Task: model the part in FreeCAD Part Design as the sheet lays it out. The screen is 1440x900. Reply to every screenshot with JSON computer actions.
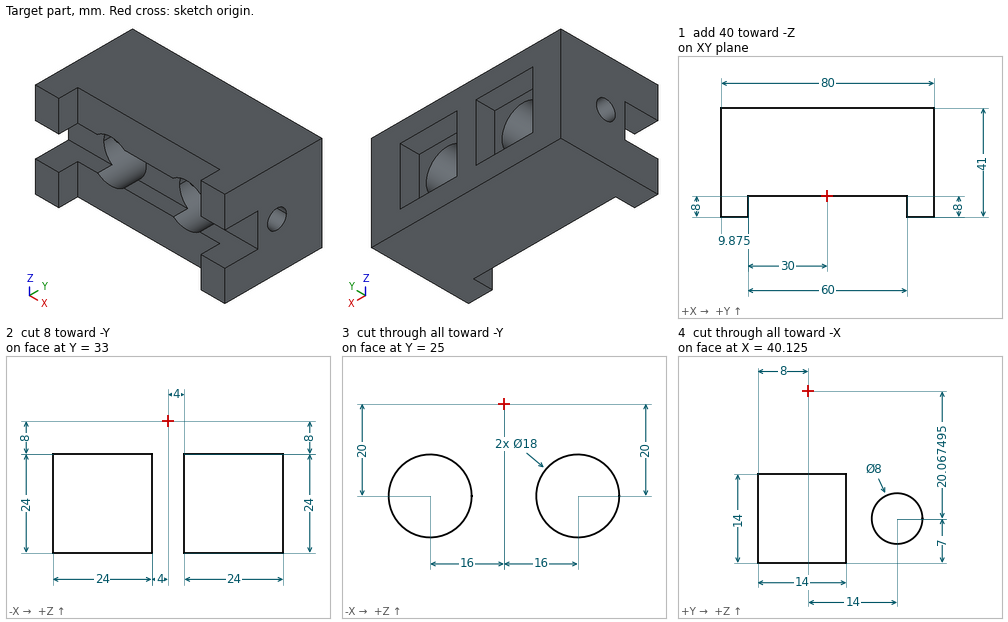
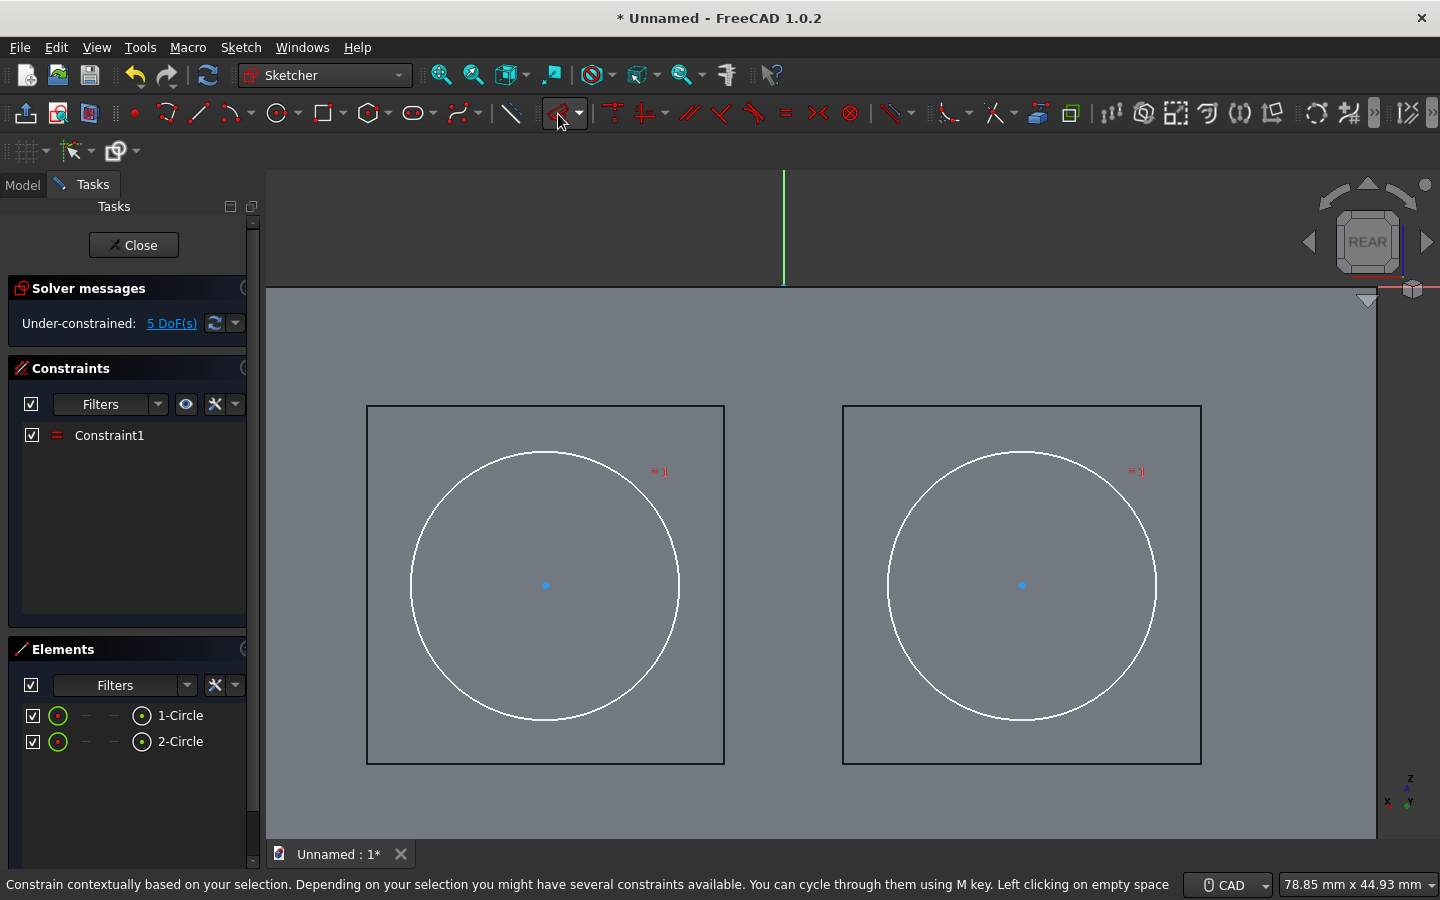
{"action": "left_click", "coordinate": [1117, 491]}
{"action": "left_click", "coordinate": [1140, 468]}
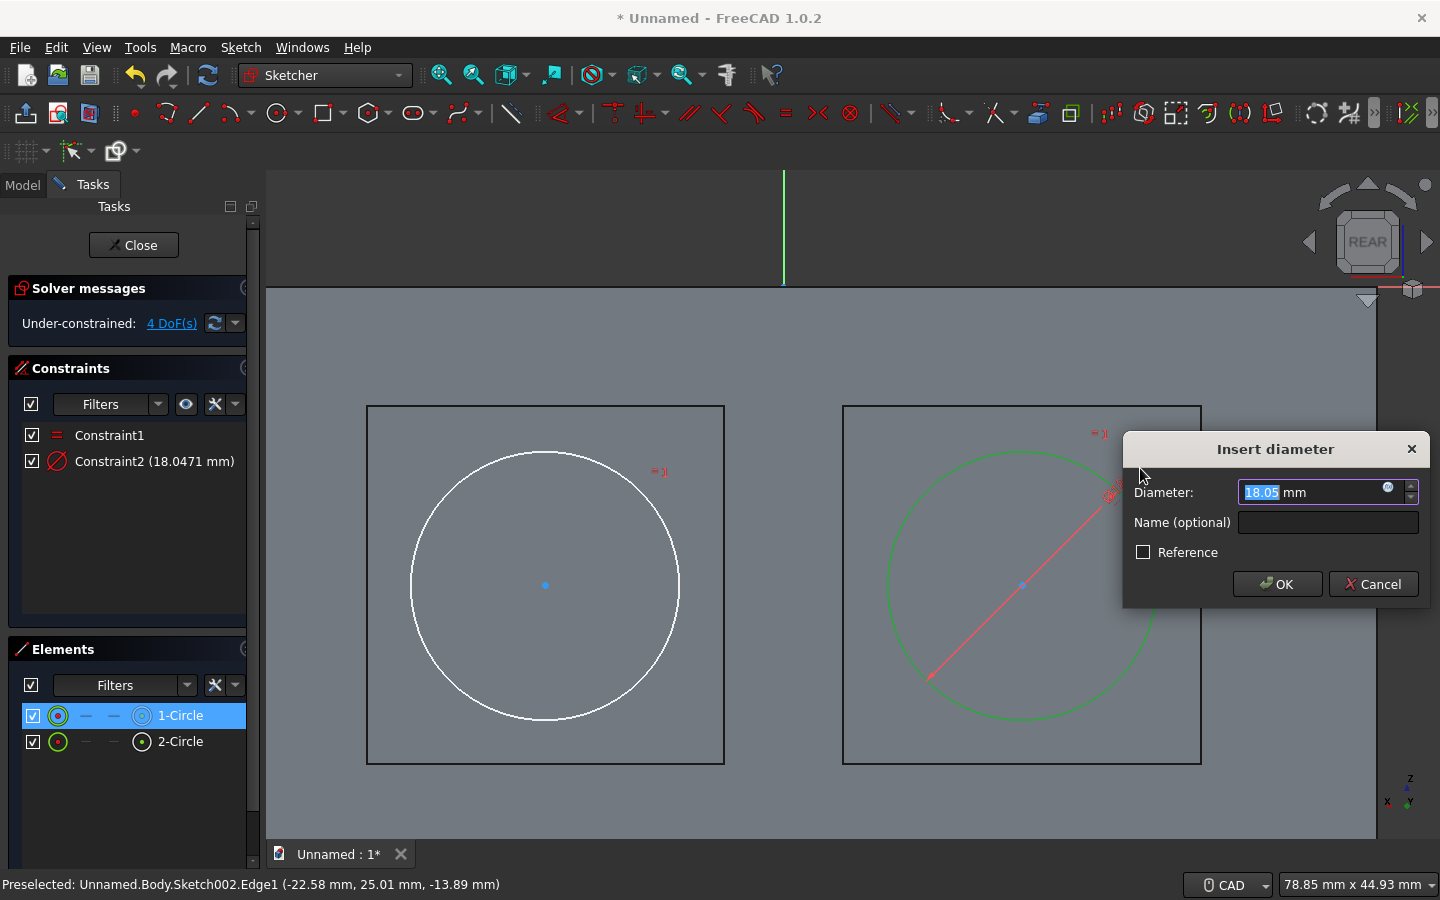
{"action": "type", "text": "18"}
{"action": "key", "text": "Return"}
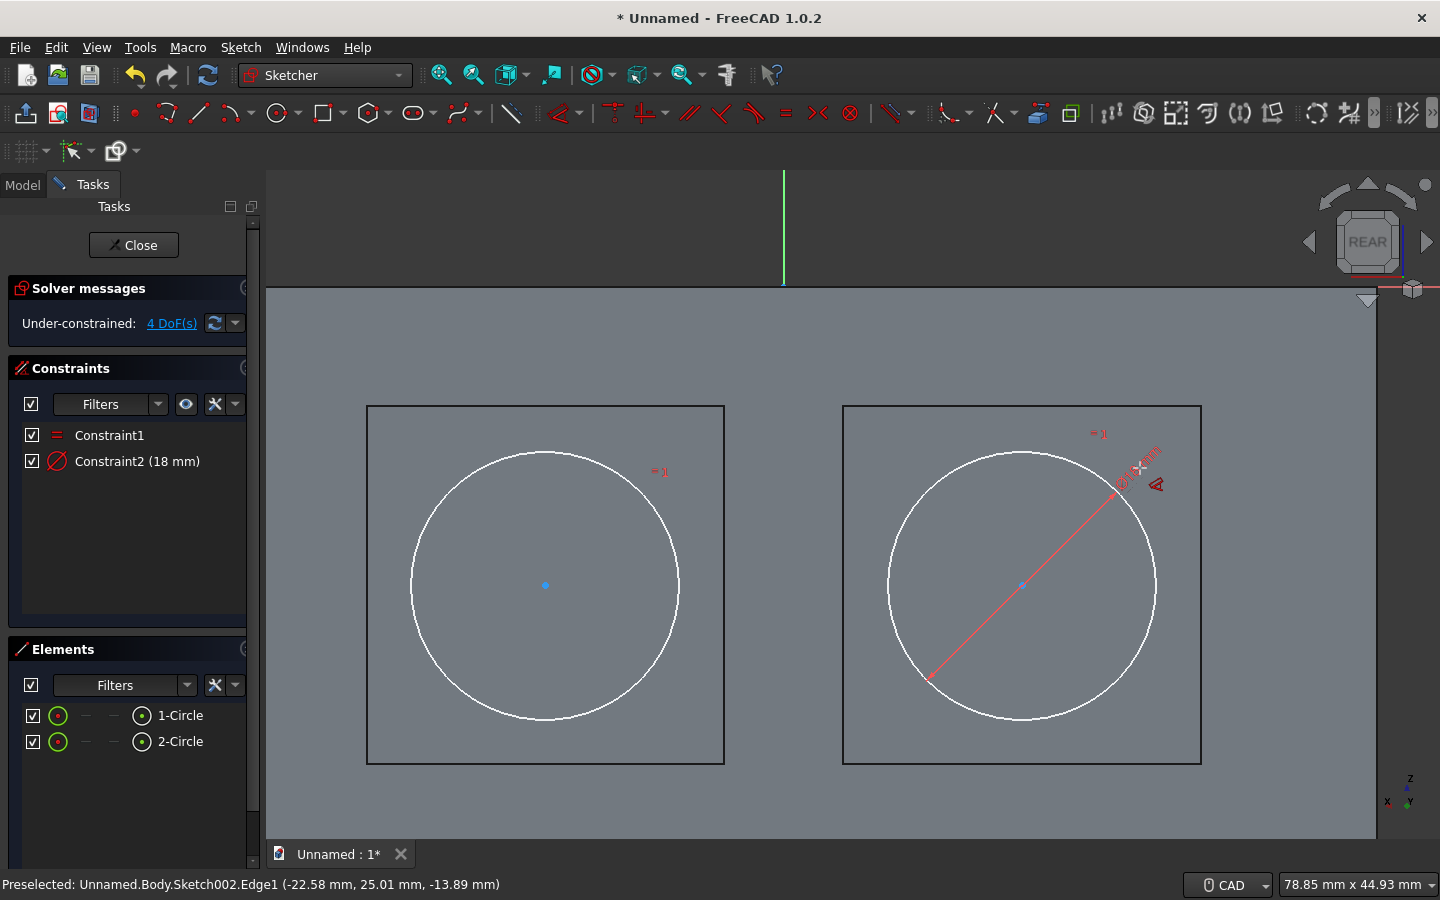
{"action": "left_click", "coordinate": [1022, 586]}
{"action": "left_click", "coordinate": [903, 253]}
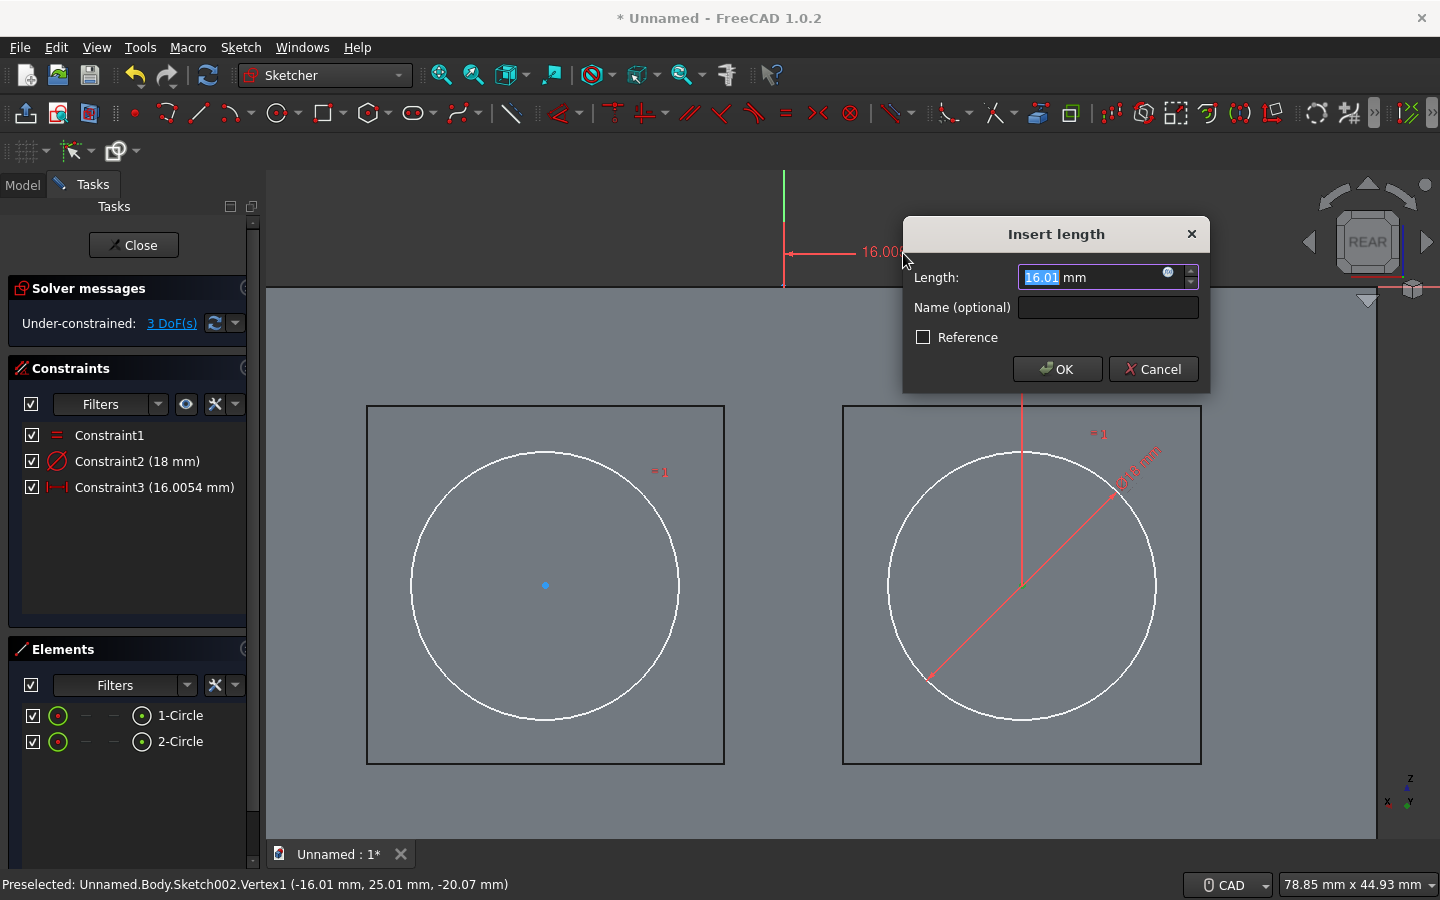
{"action": "type", "text": "16"}
{"action": "key", "text": "Return"}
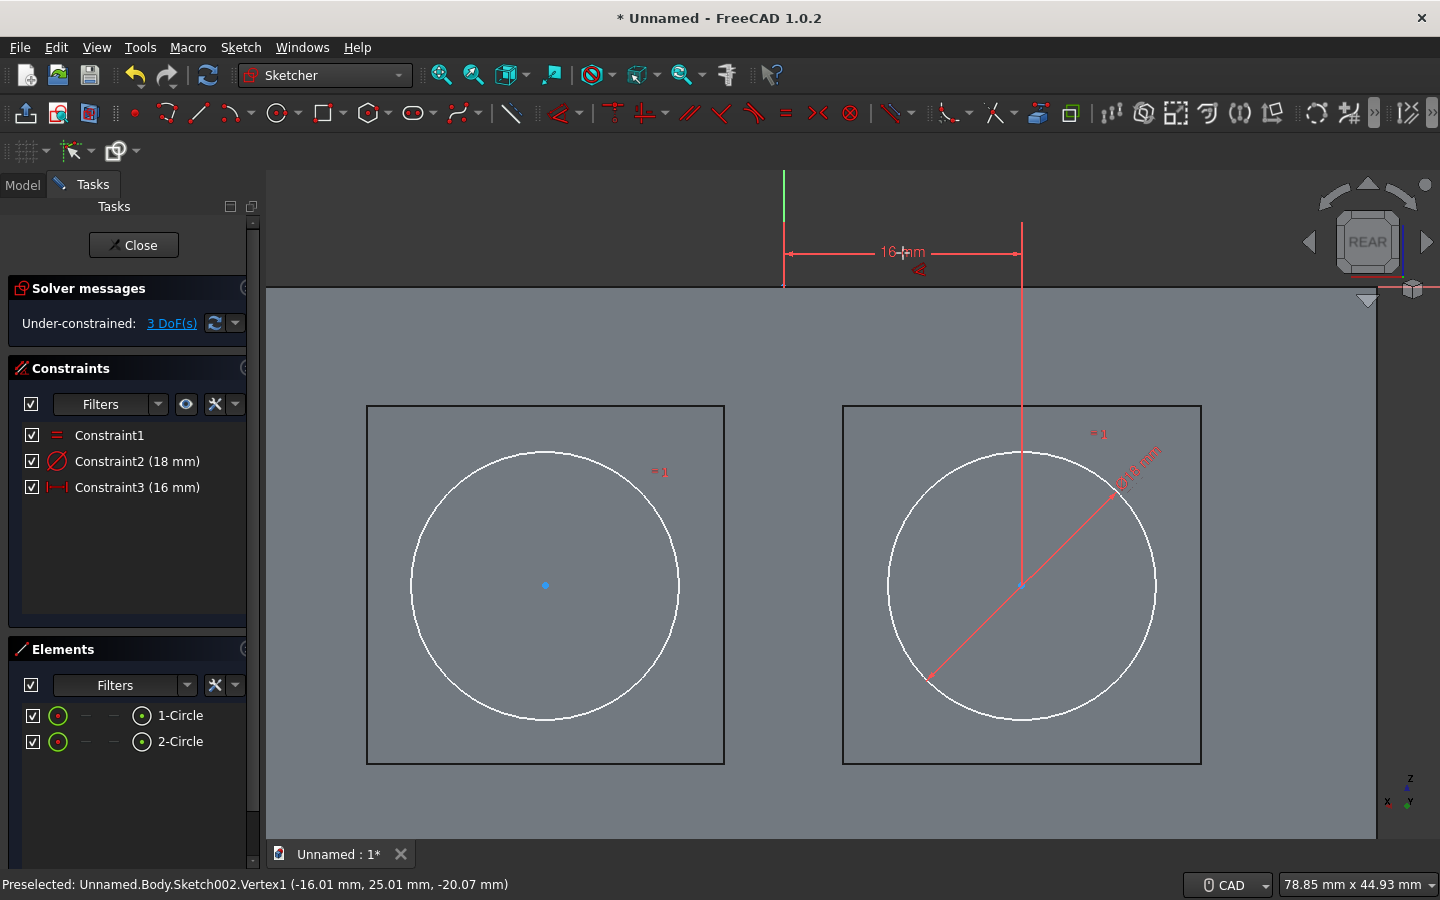
{"action": "left_click", "coordinate": [1022, 586]}
{"action": "left_click", "coordinate": [1056, 437]}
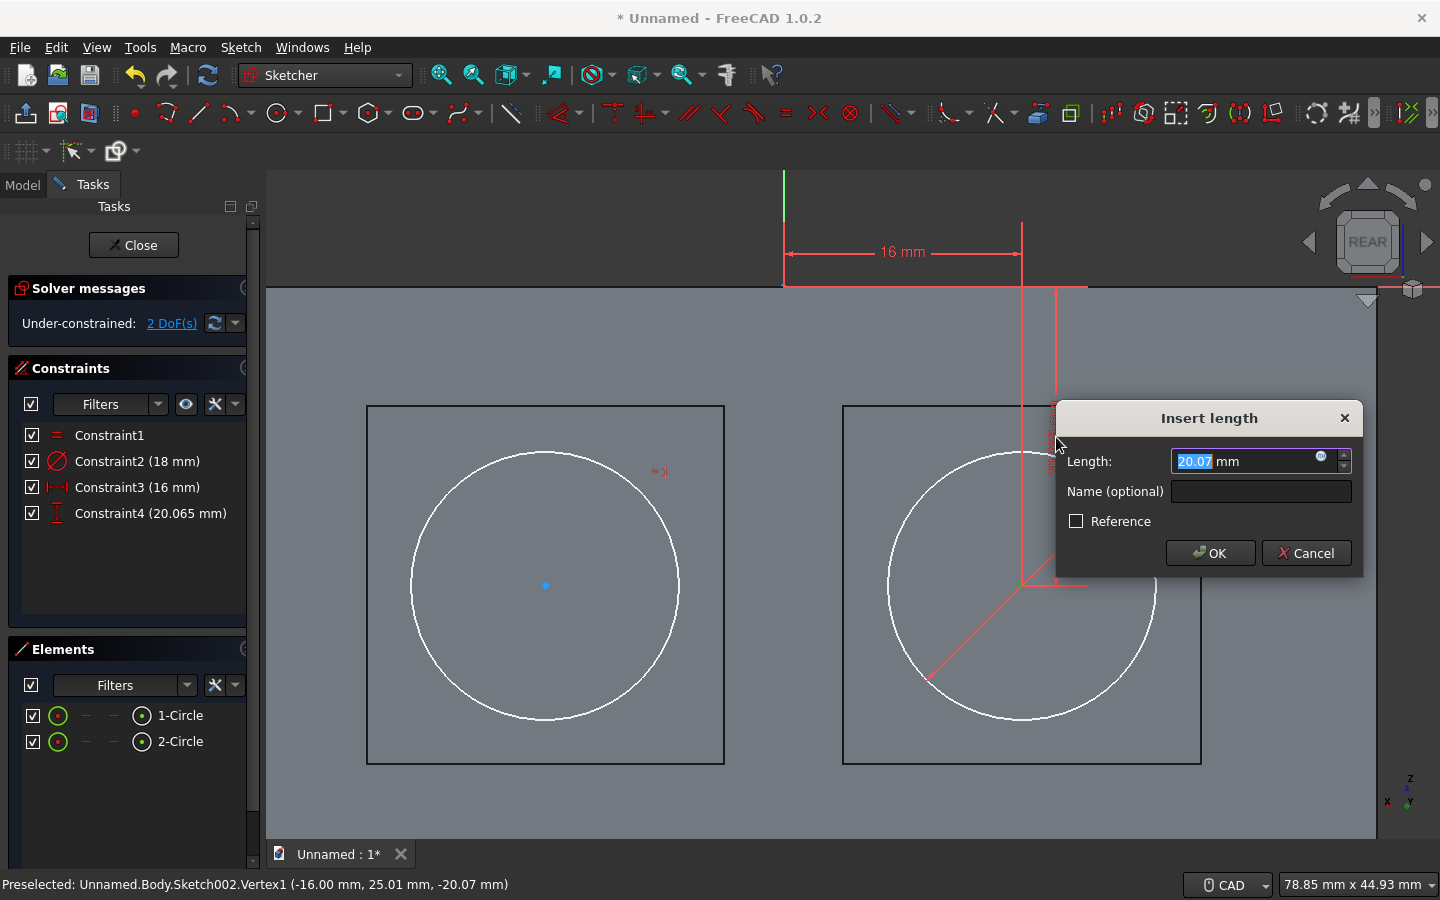
{"action": "type", "text": "20"}
{"action": "key", "text": "Return"}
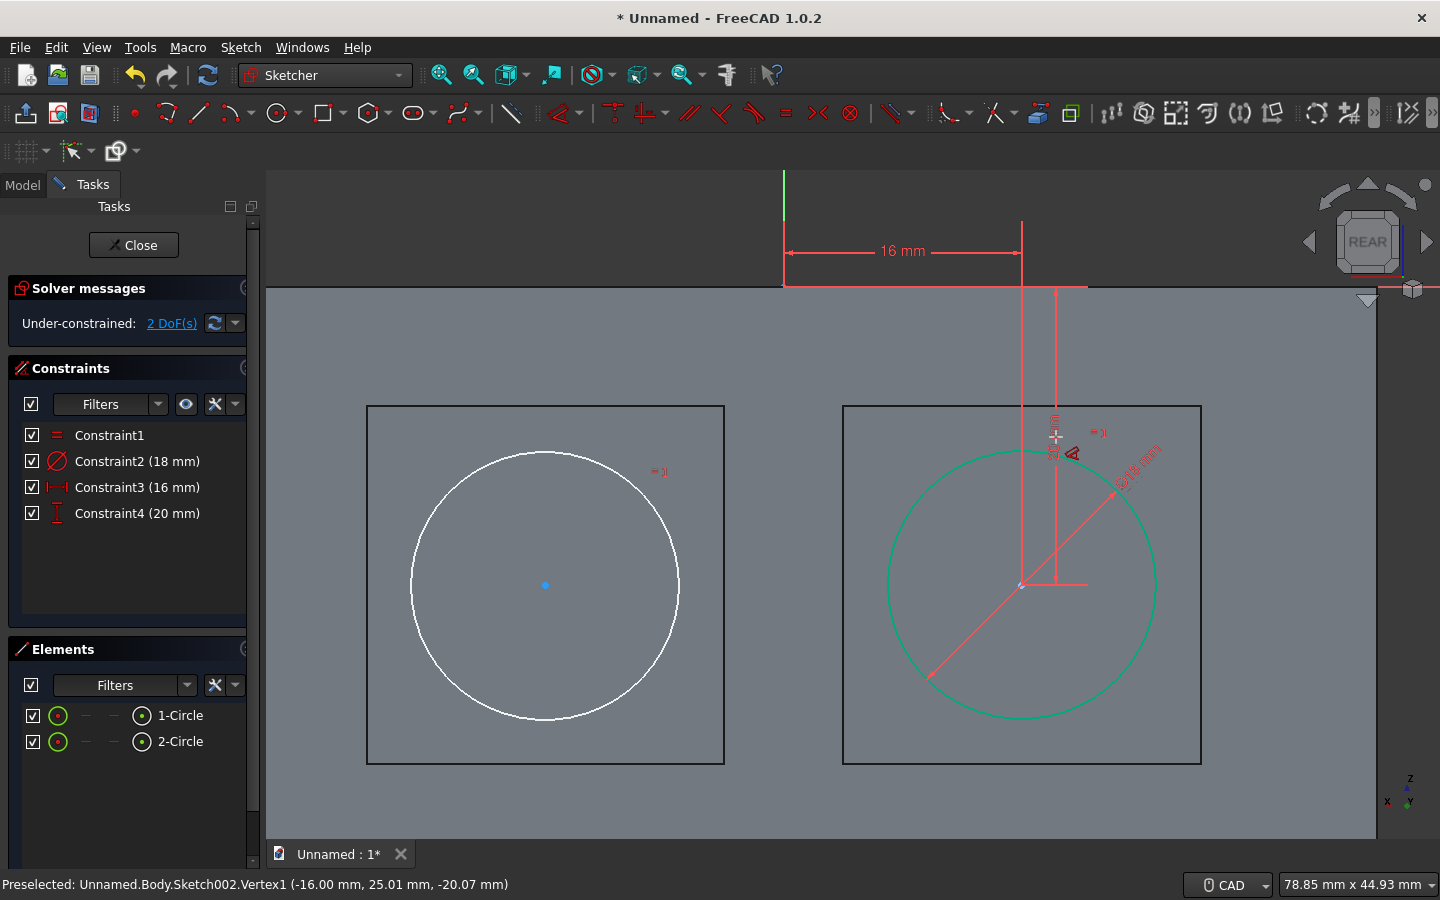
{"action": "left_click", "coordinate": [545, 586]}
{"action": "left_click", "coordinate": [664, 253]}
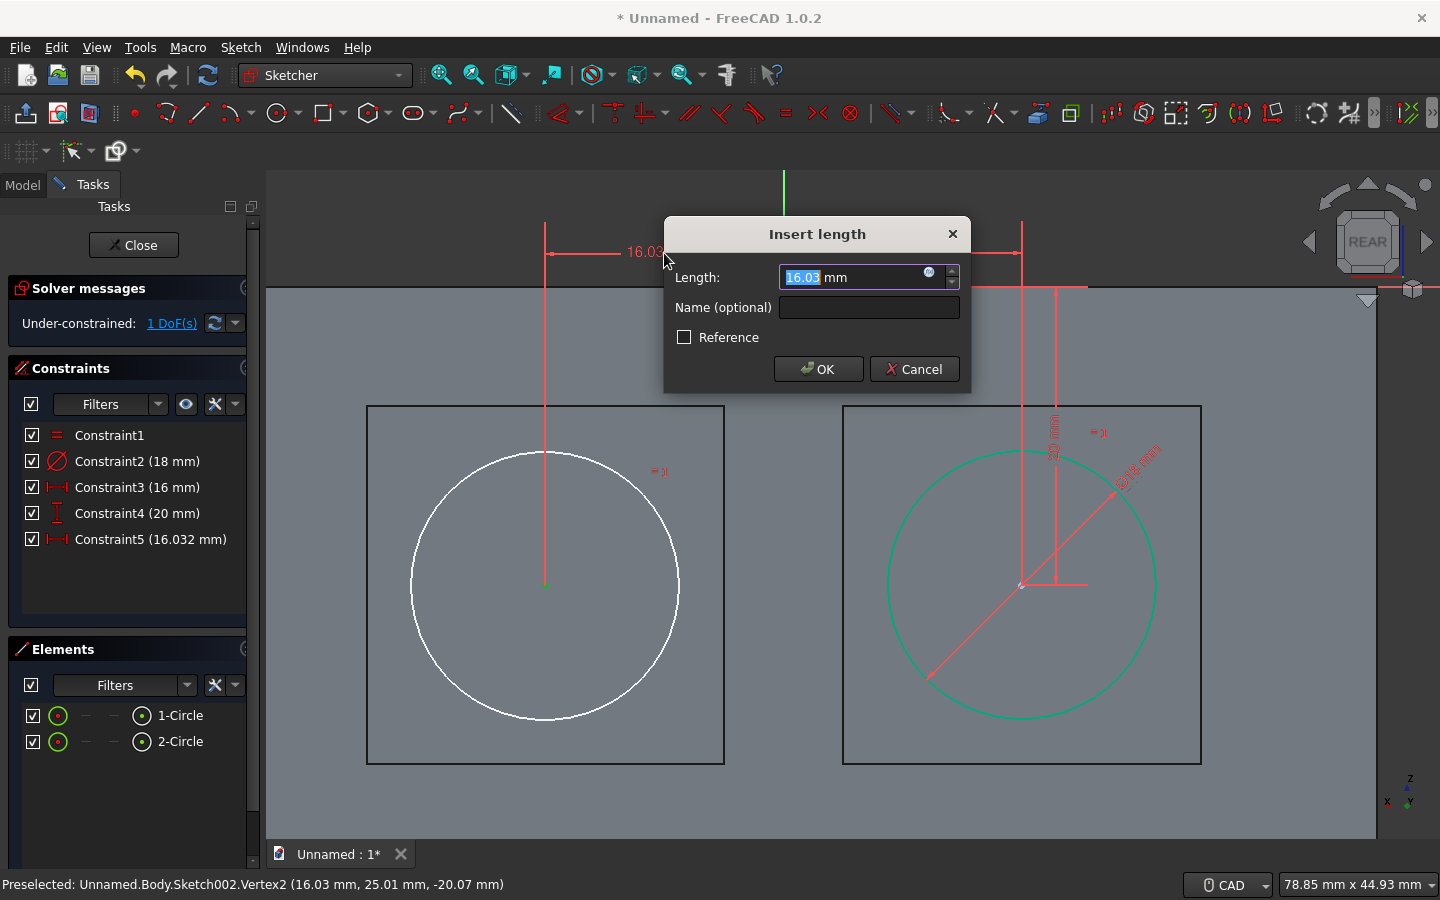
{"action": "type", "text": "16"}
{"action": "key", "text": "Return"}